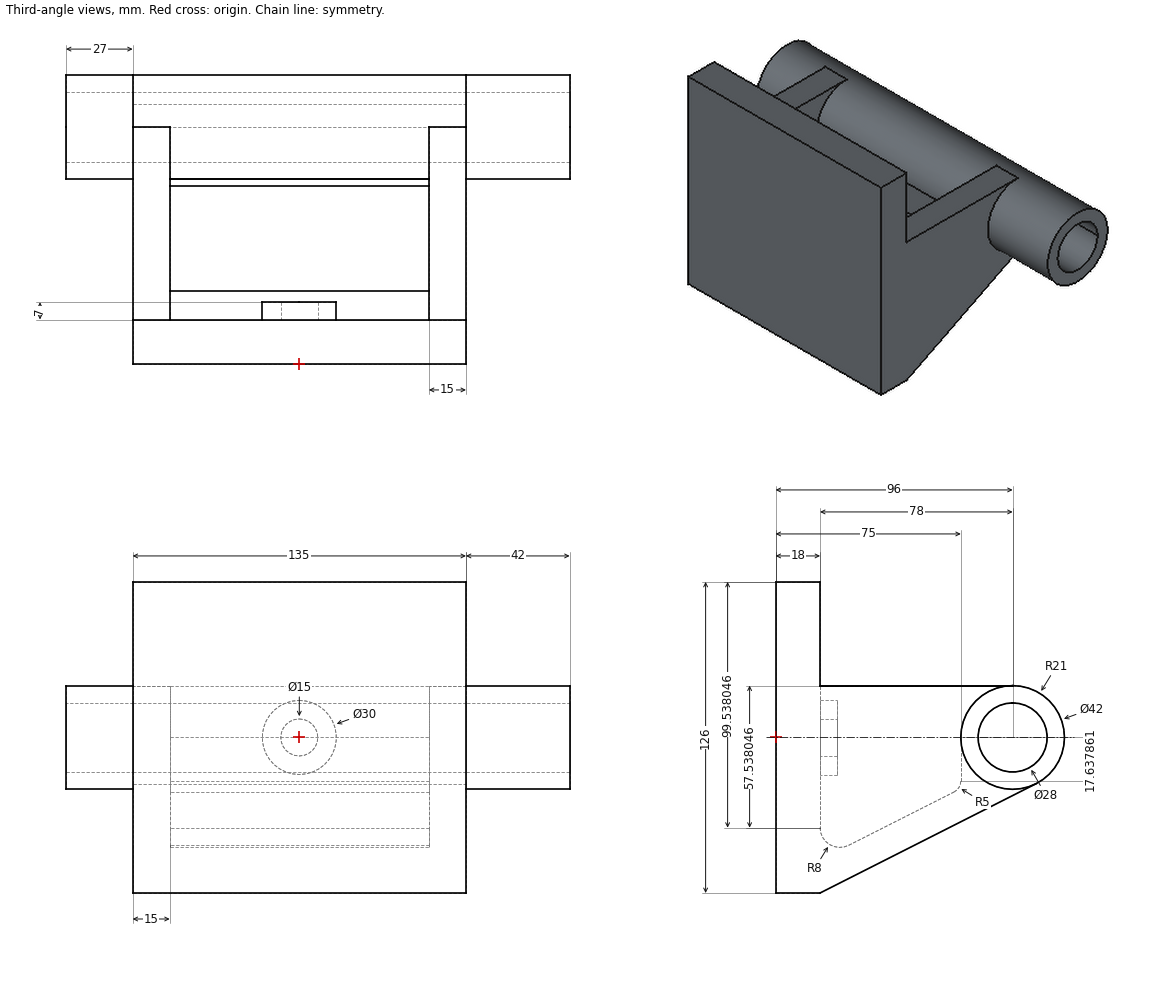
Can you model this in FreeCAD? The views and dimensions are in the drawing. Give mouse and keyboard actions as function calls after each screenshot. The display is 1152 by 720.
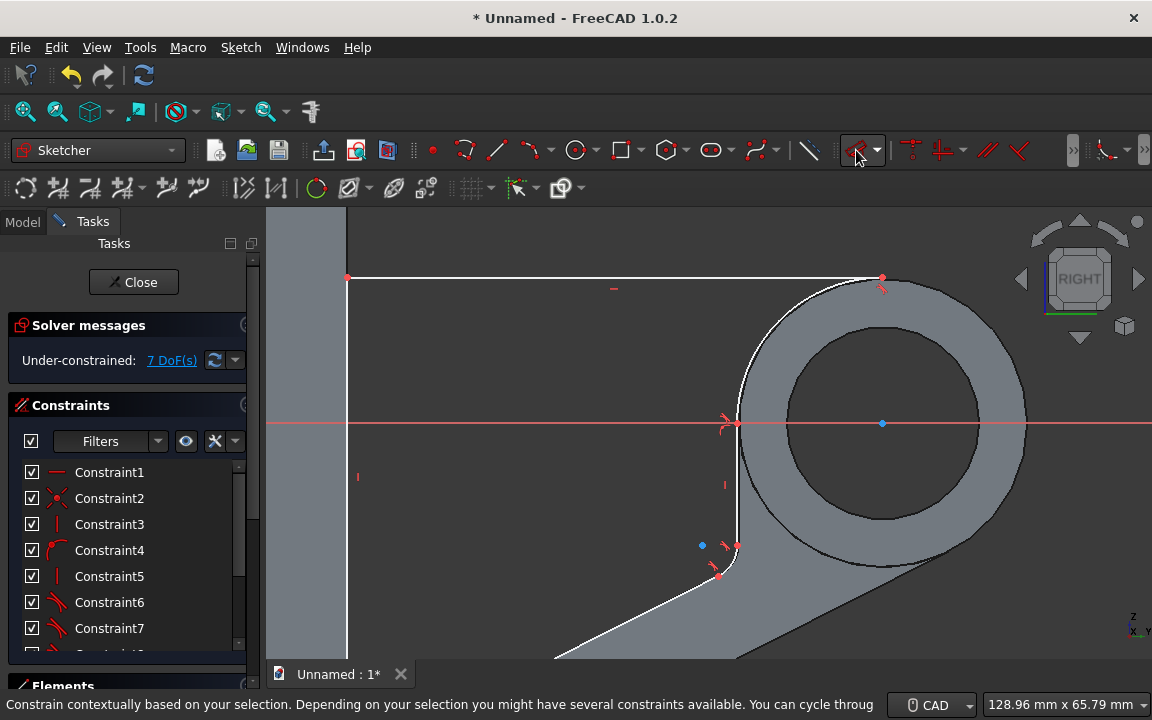
scroll(818, 295, down, 2)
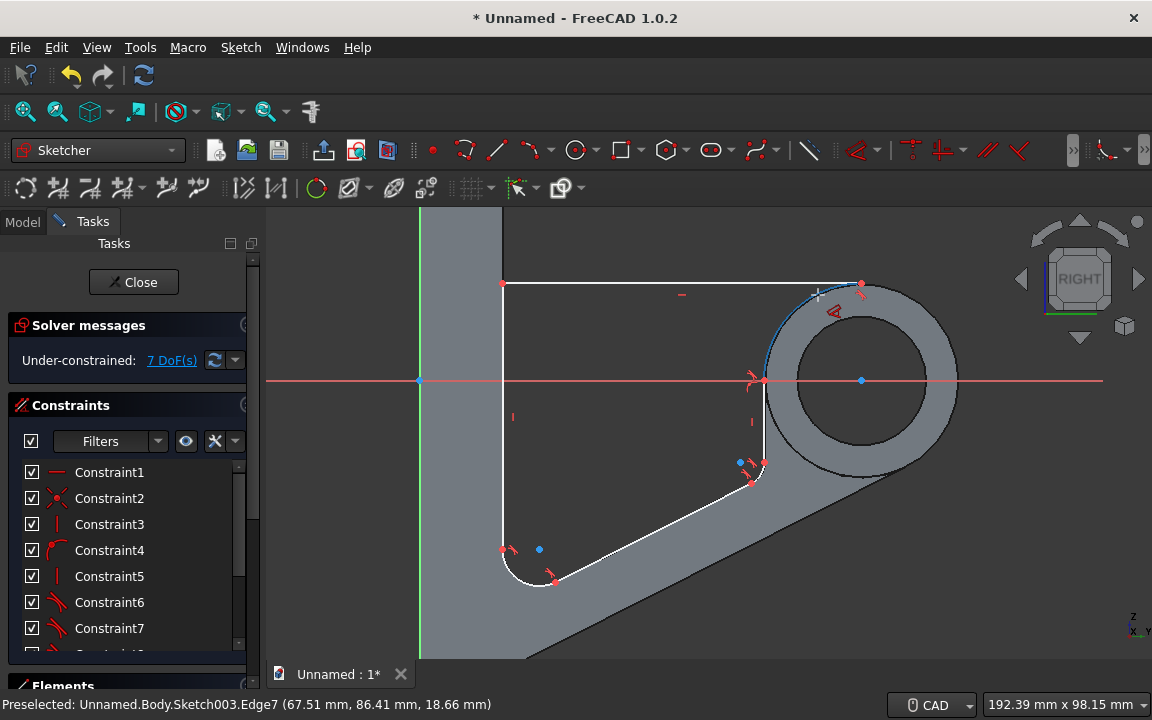
click(509, 570)
click(483, 588)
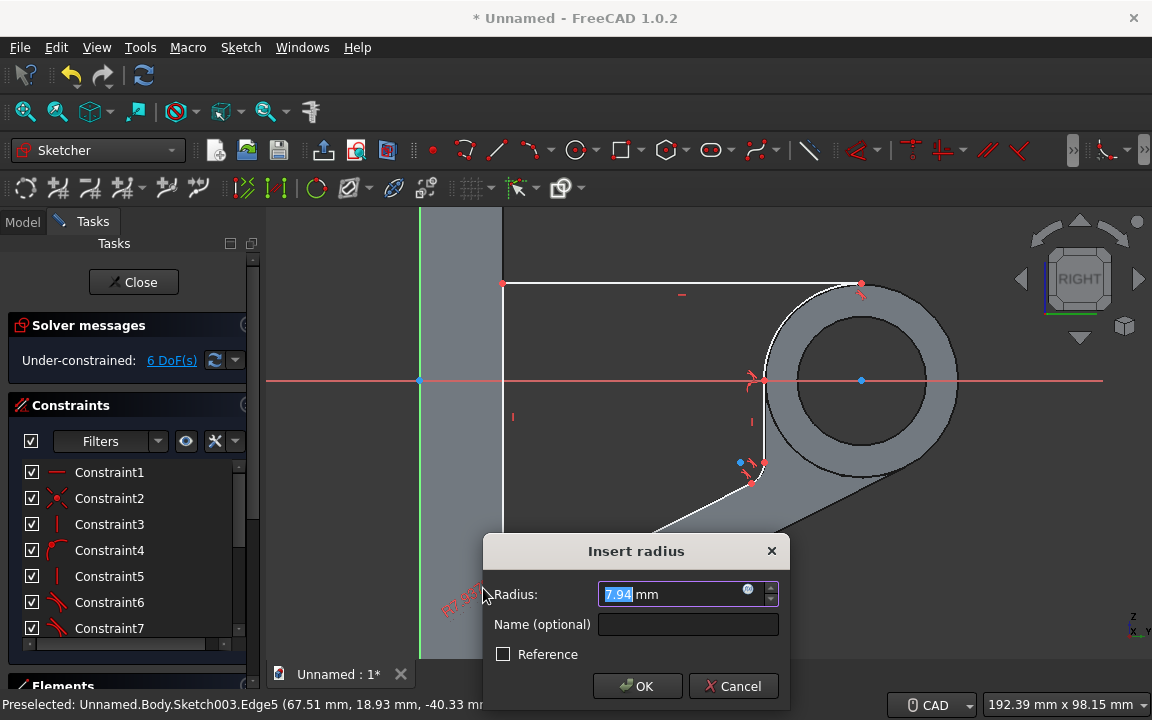
text(8)
key(Return)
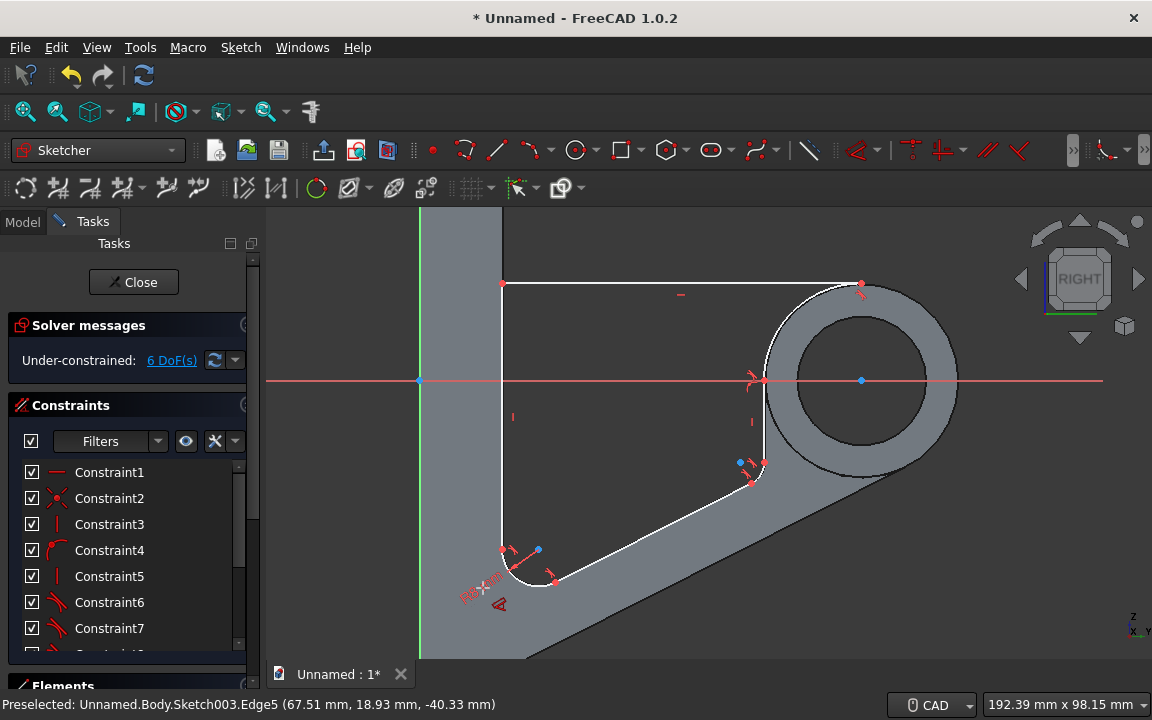
scroll(761, 475, up, 3)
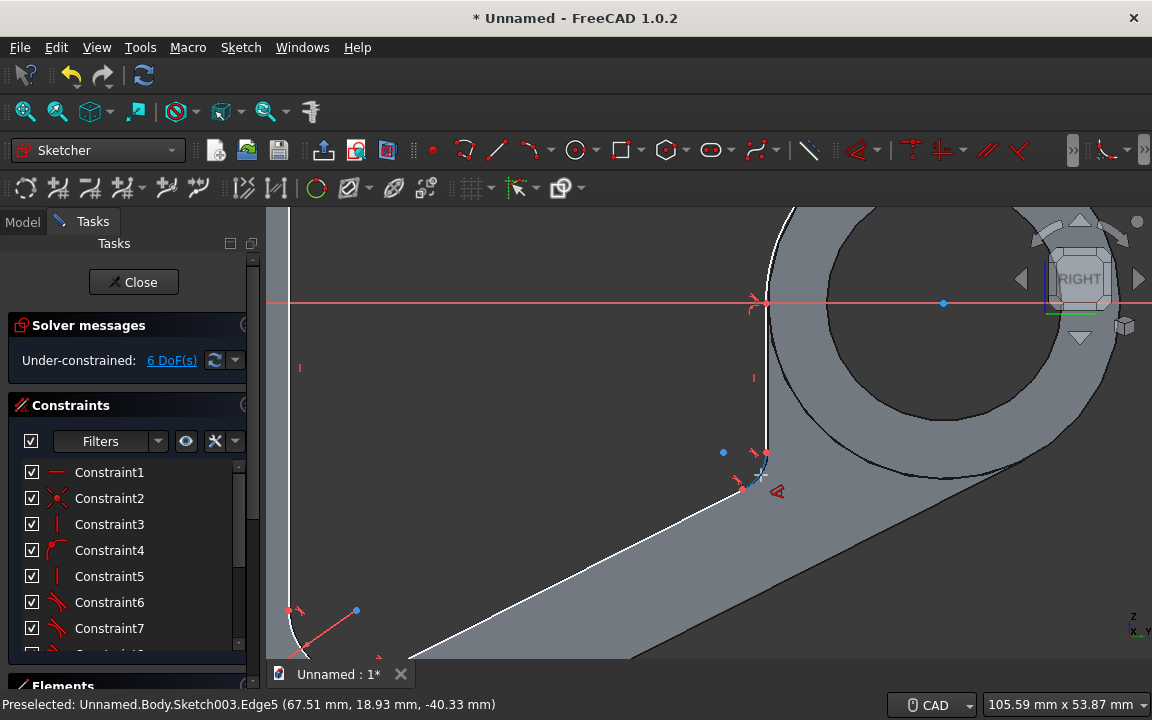
click(760, 474)
click(787, 490)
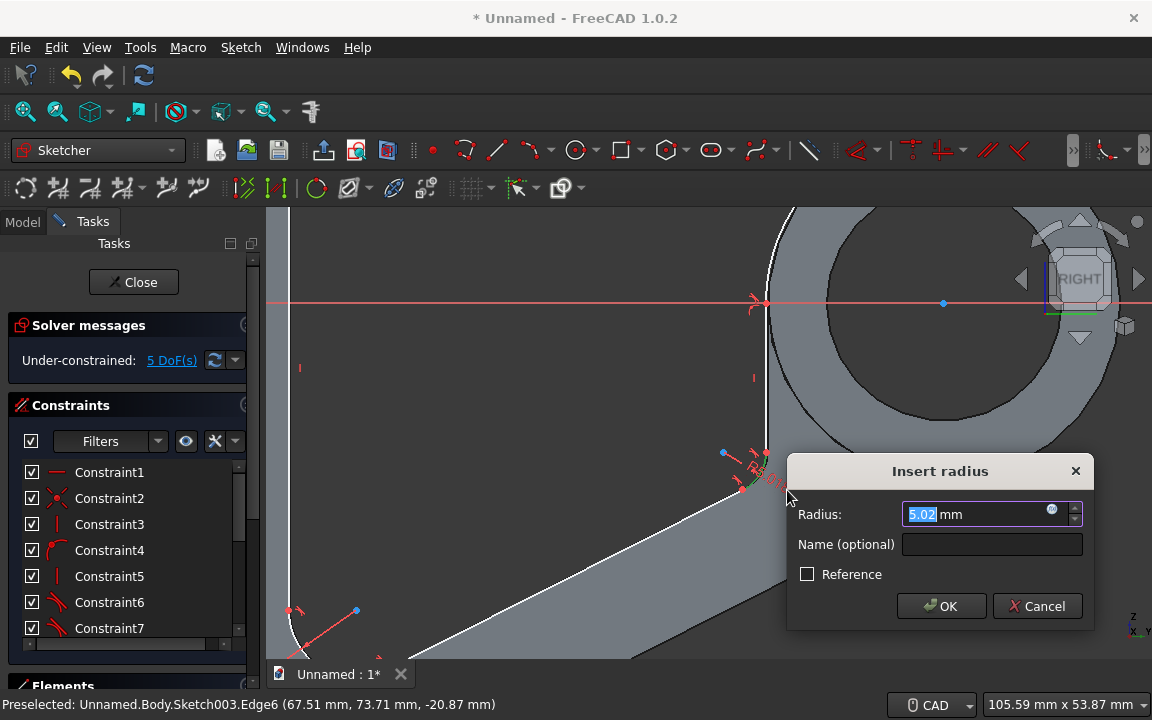
text(5)
key(Return)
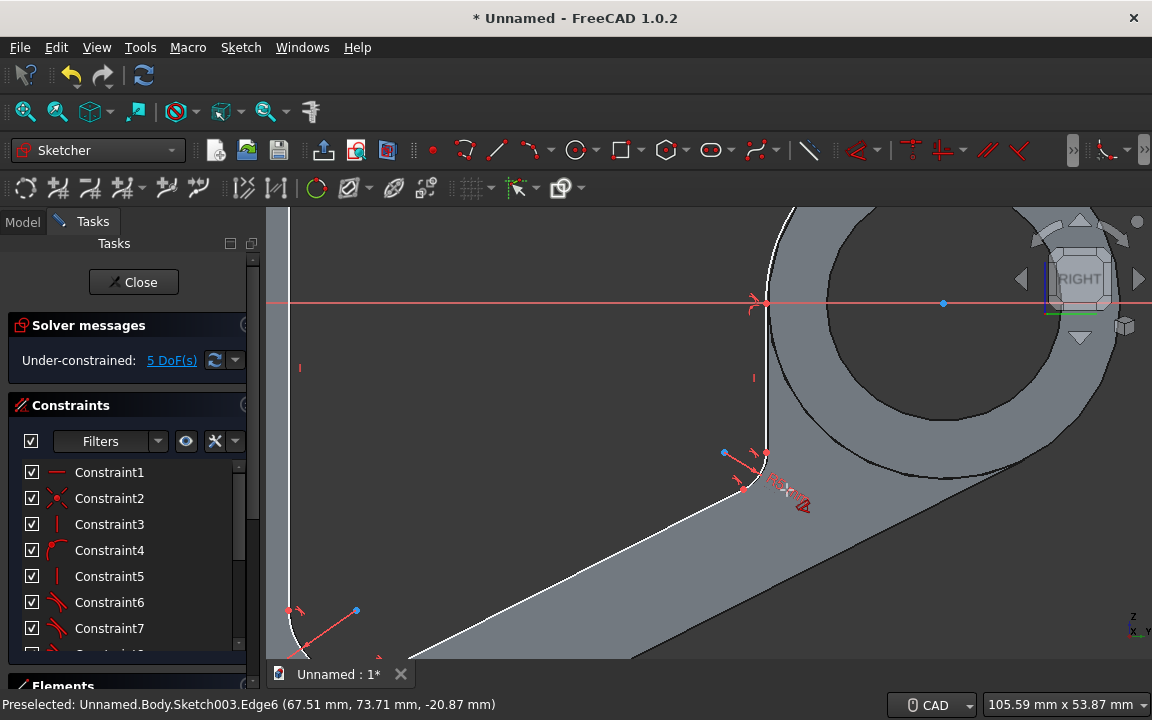
click(775, 248)
click(745, 238)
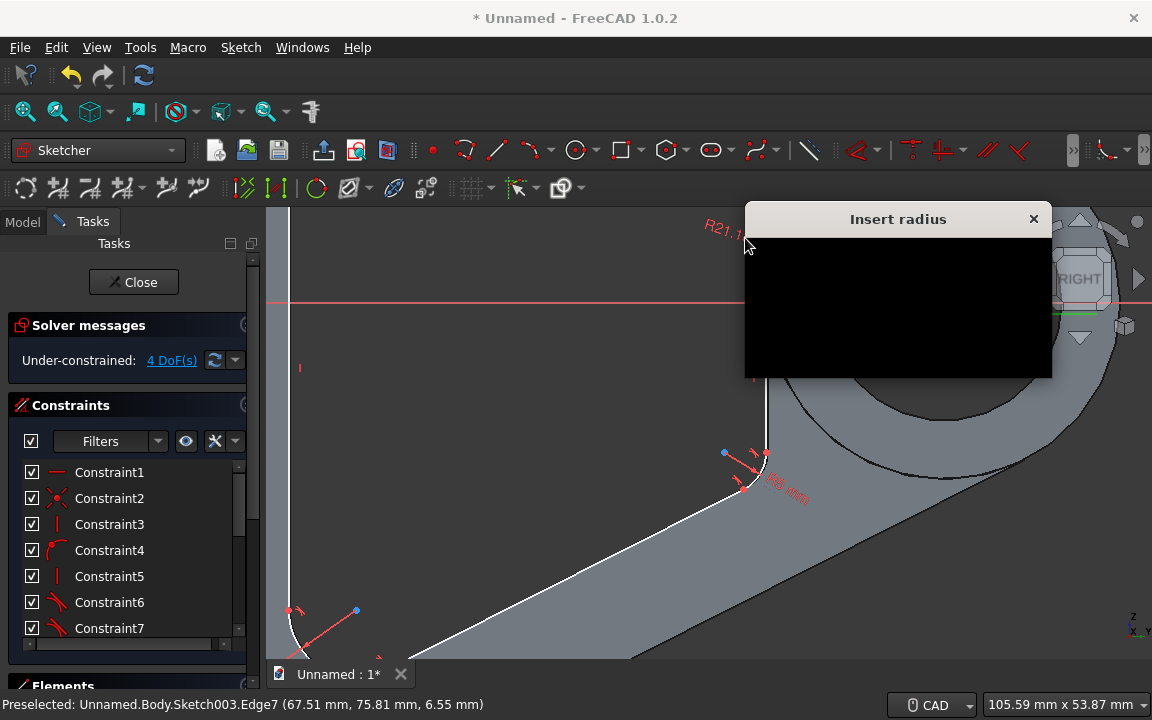
text(21)
key(Return)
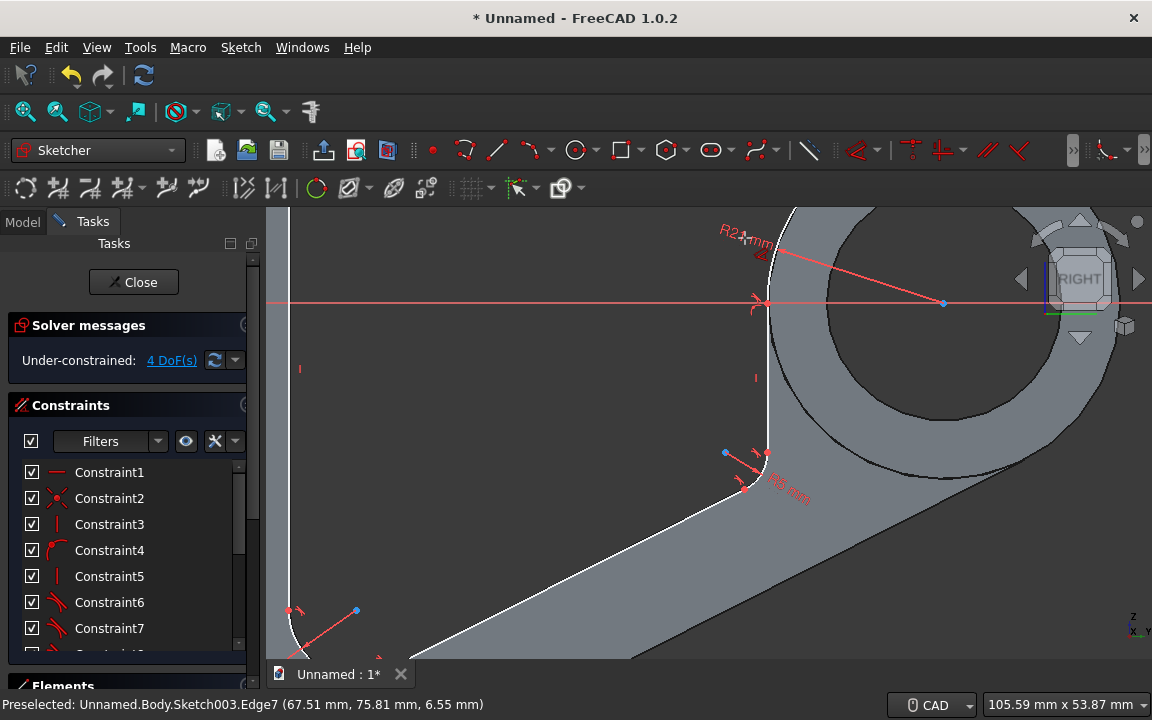
scroll(761, 475, down, 3)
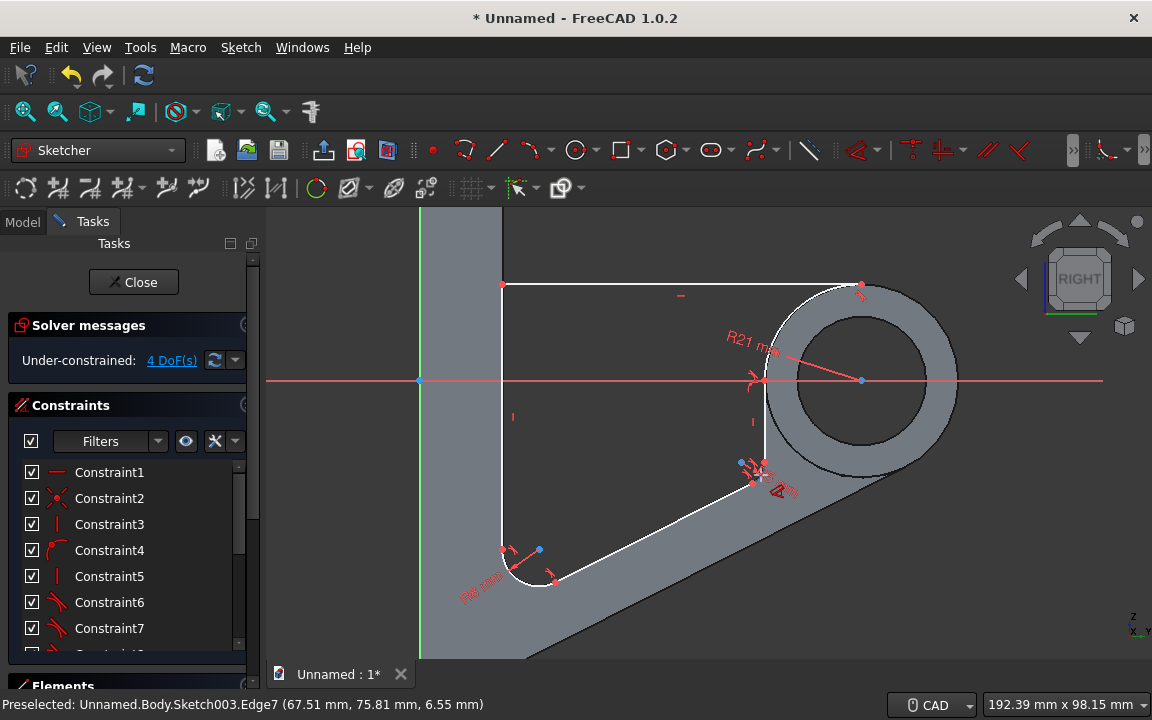
click(754, 284)
click(682, 250)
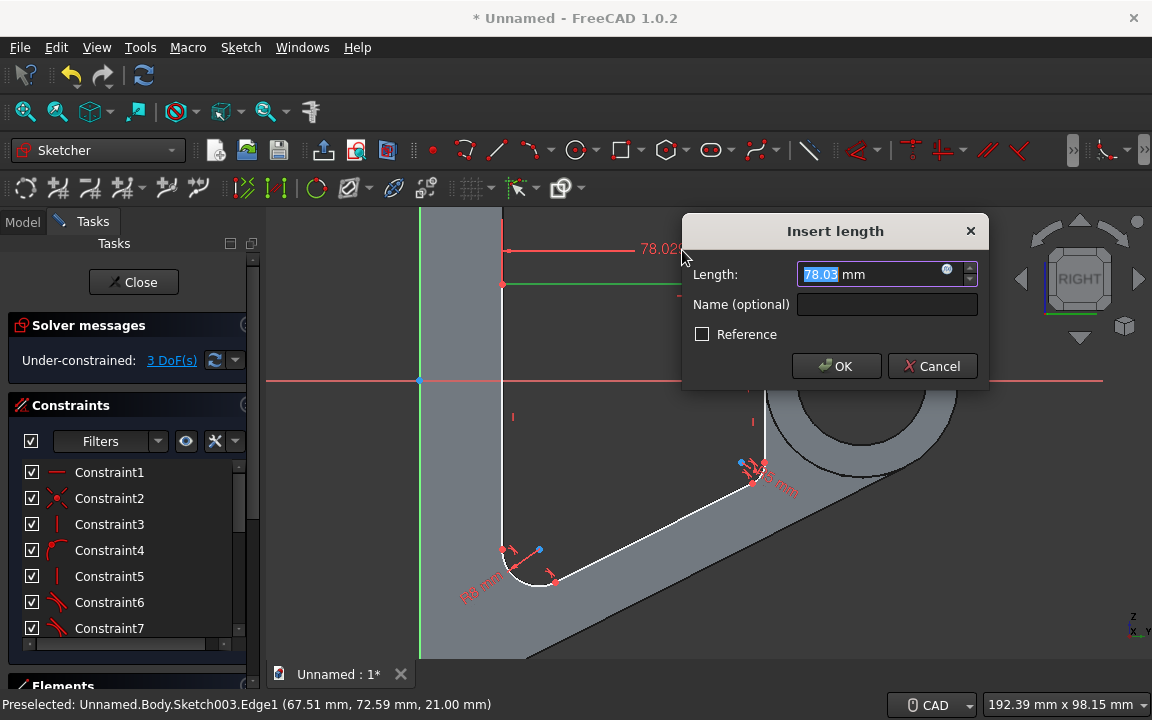
text(78)
key(Return)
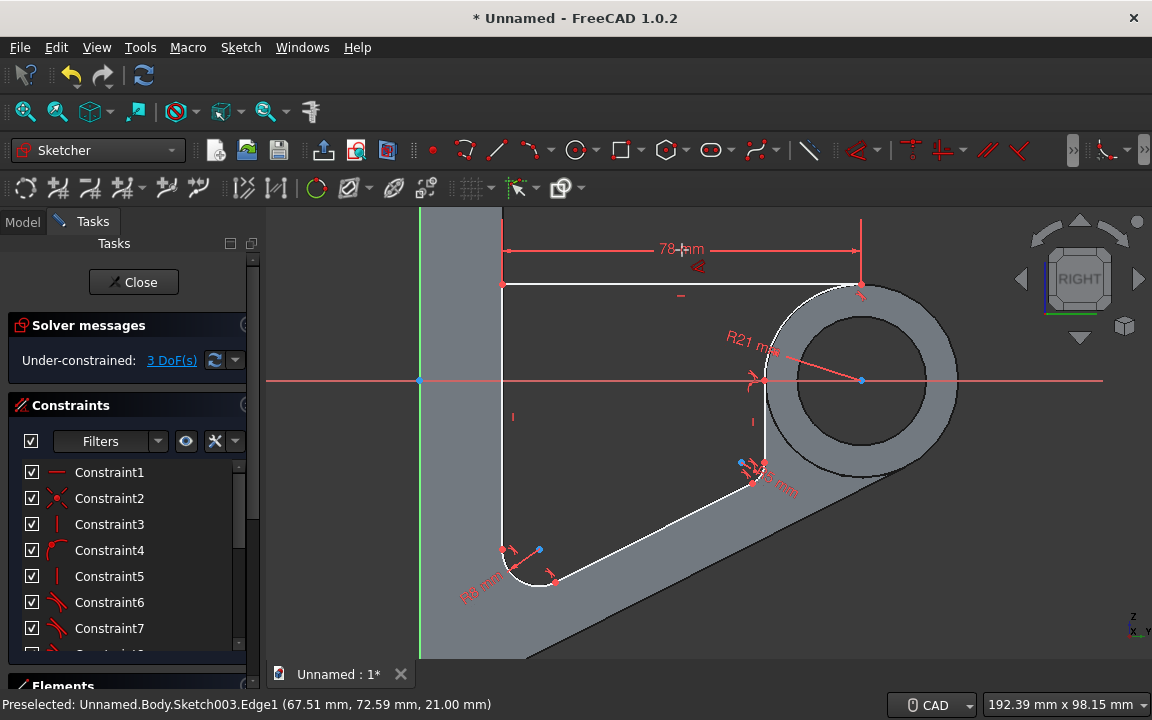
click(861, 284)
click(539, 250)